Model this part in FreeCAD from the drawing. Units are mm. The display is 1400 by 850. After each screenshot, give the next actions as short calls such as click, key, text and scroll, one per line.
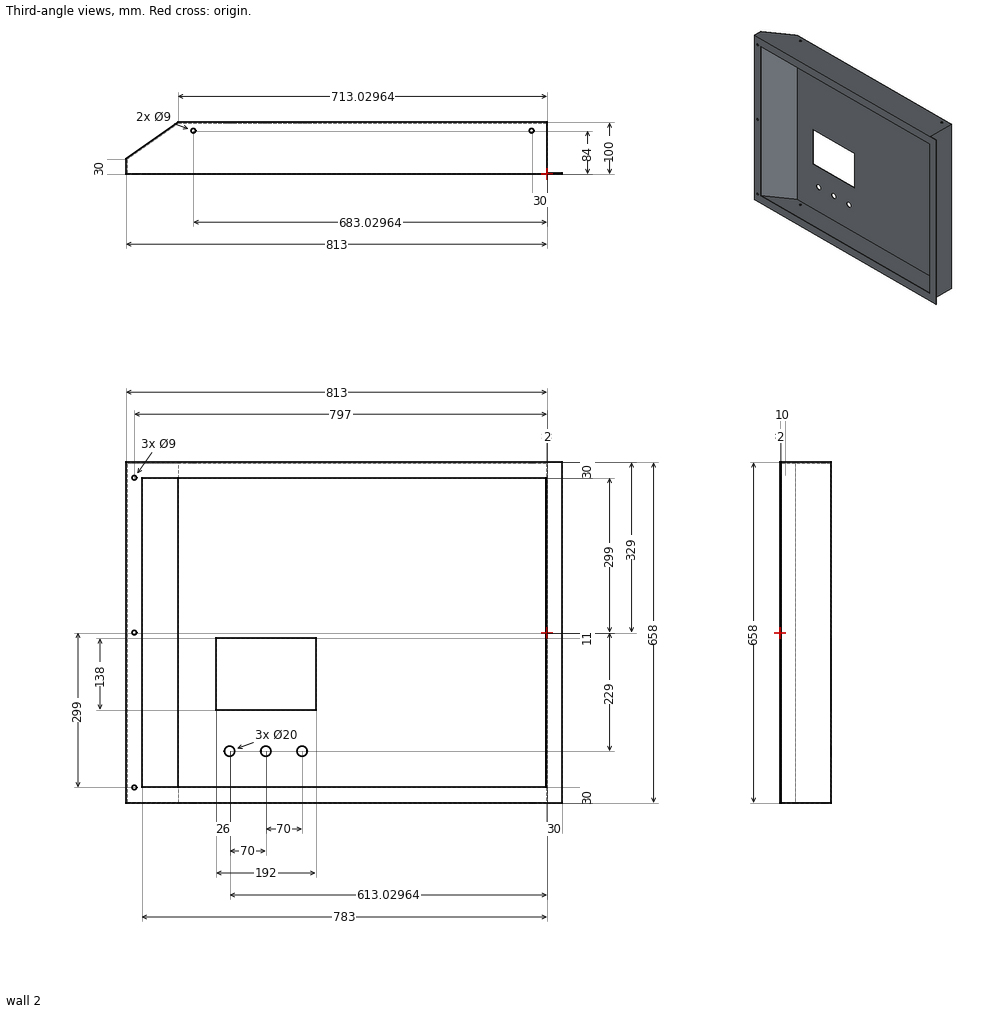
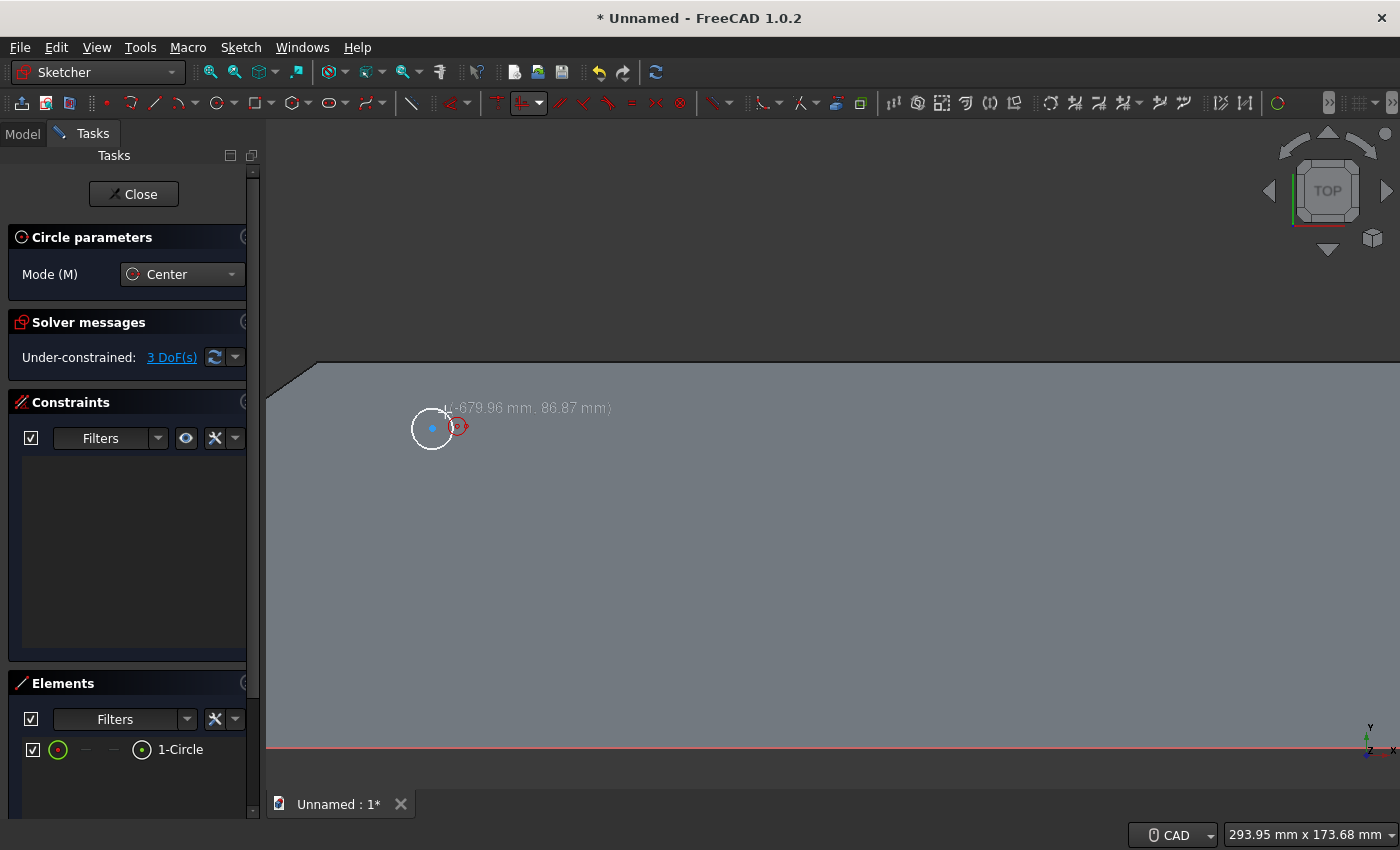
scroll(445, 414, down, 7)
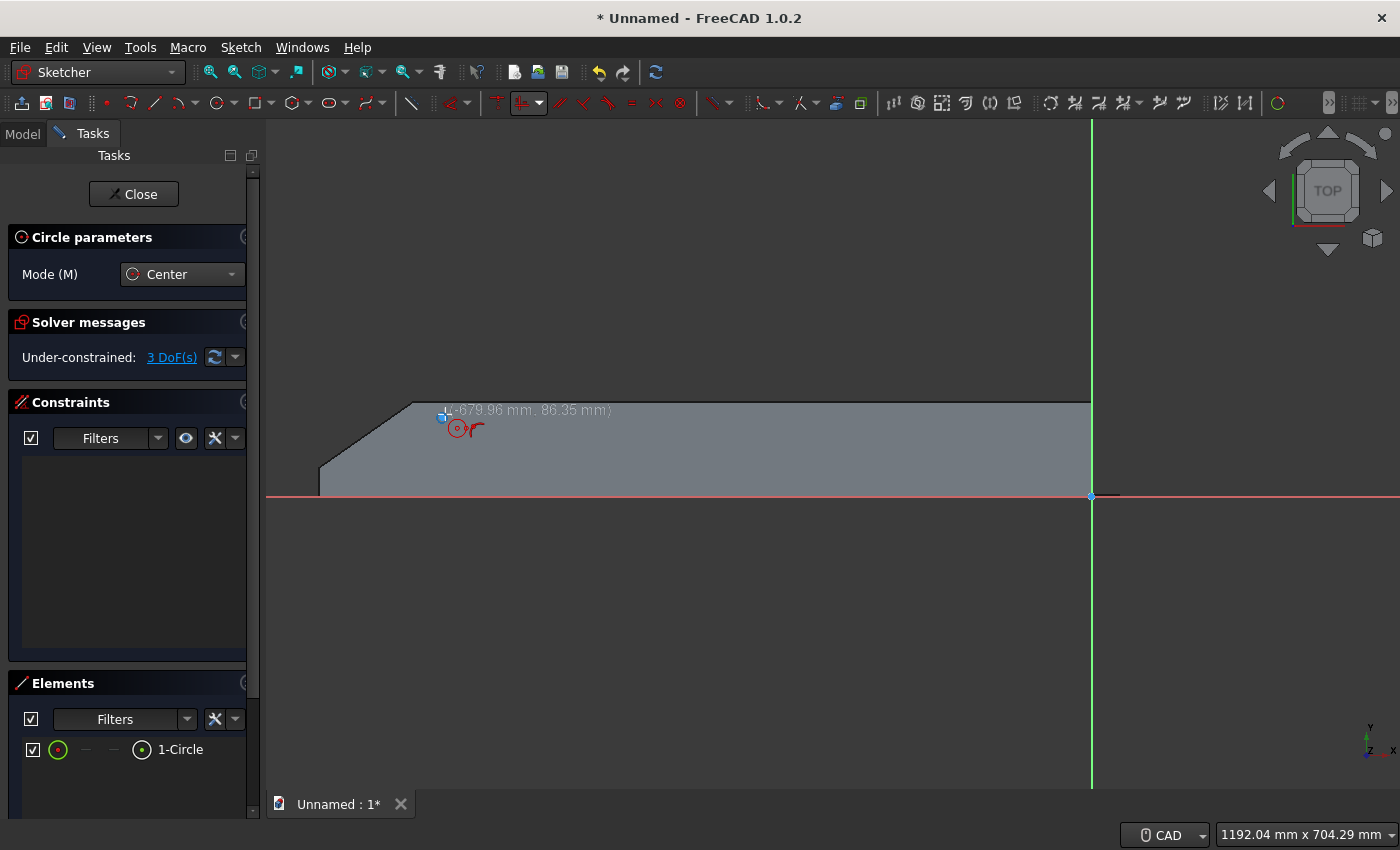
scroll(1063, 417, up, 9)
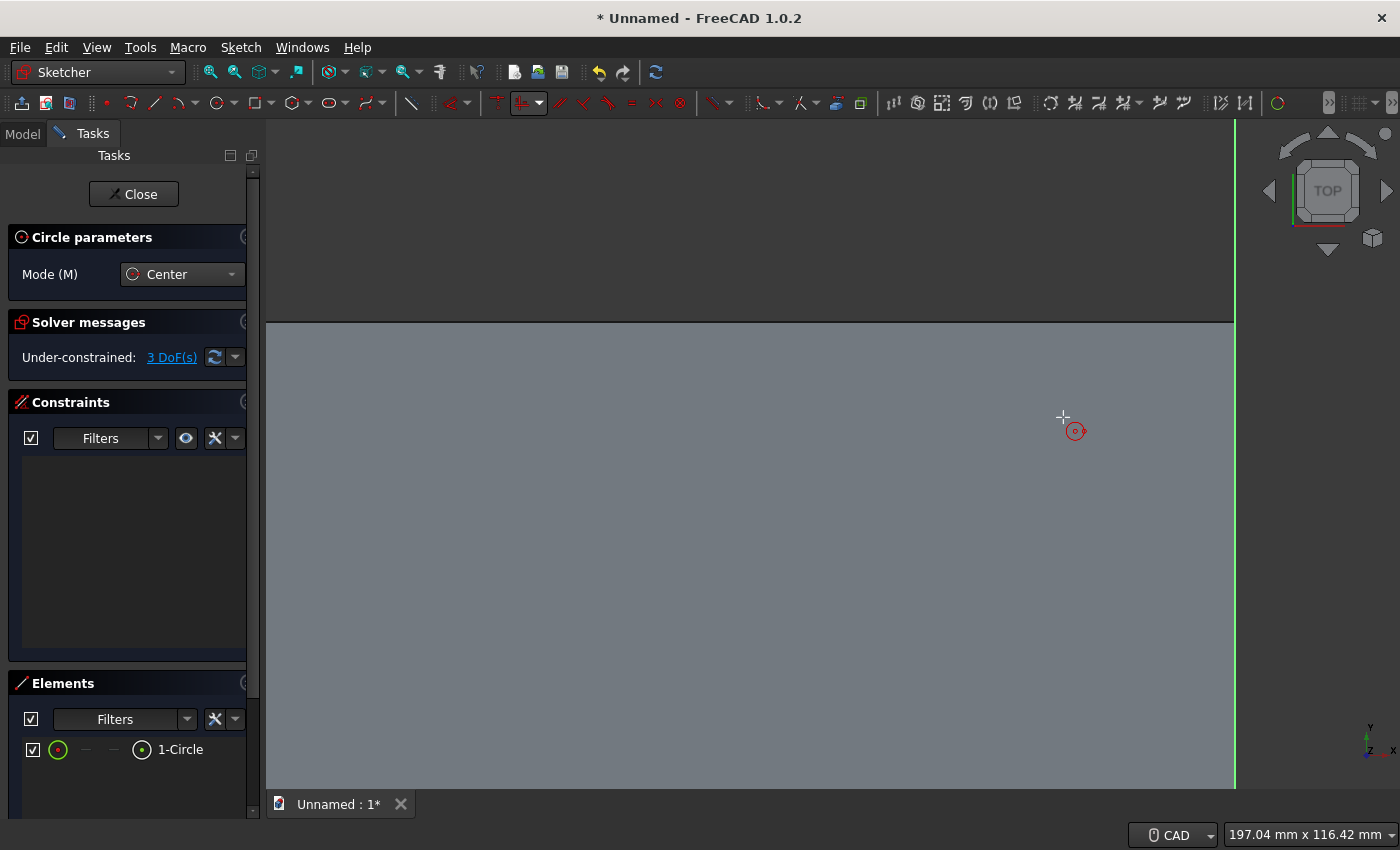
scroll(1063, 417, down, 9)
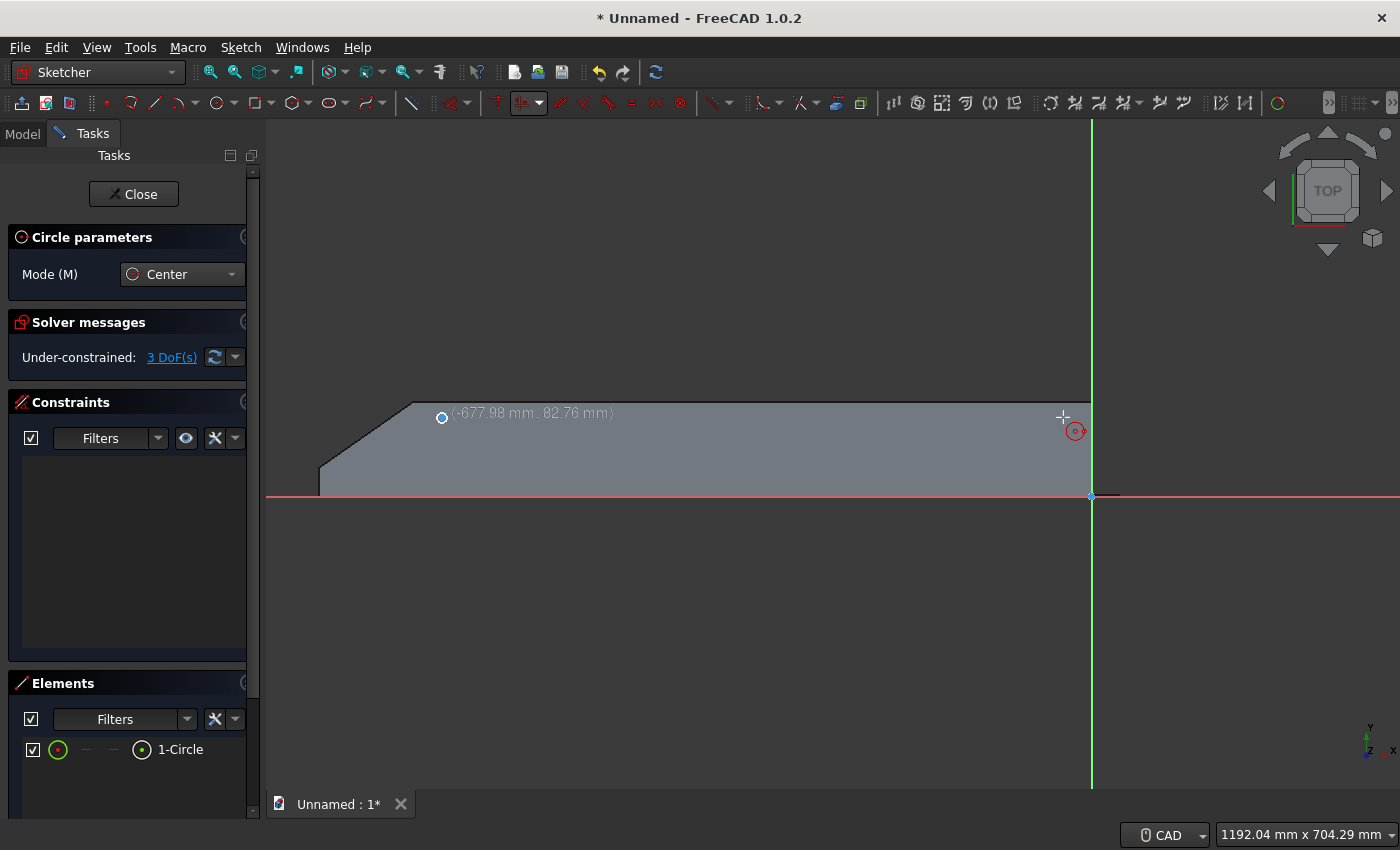
click(1063, 417)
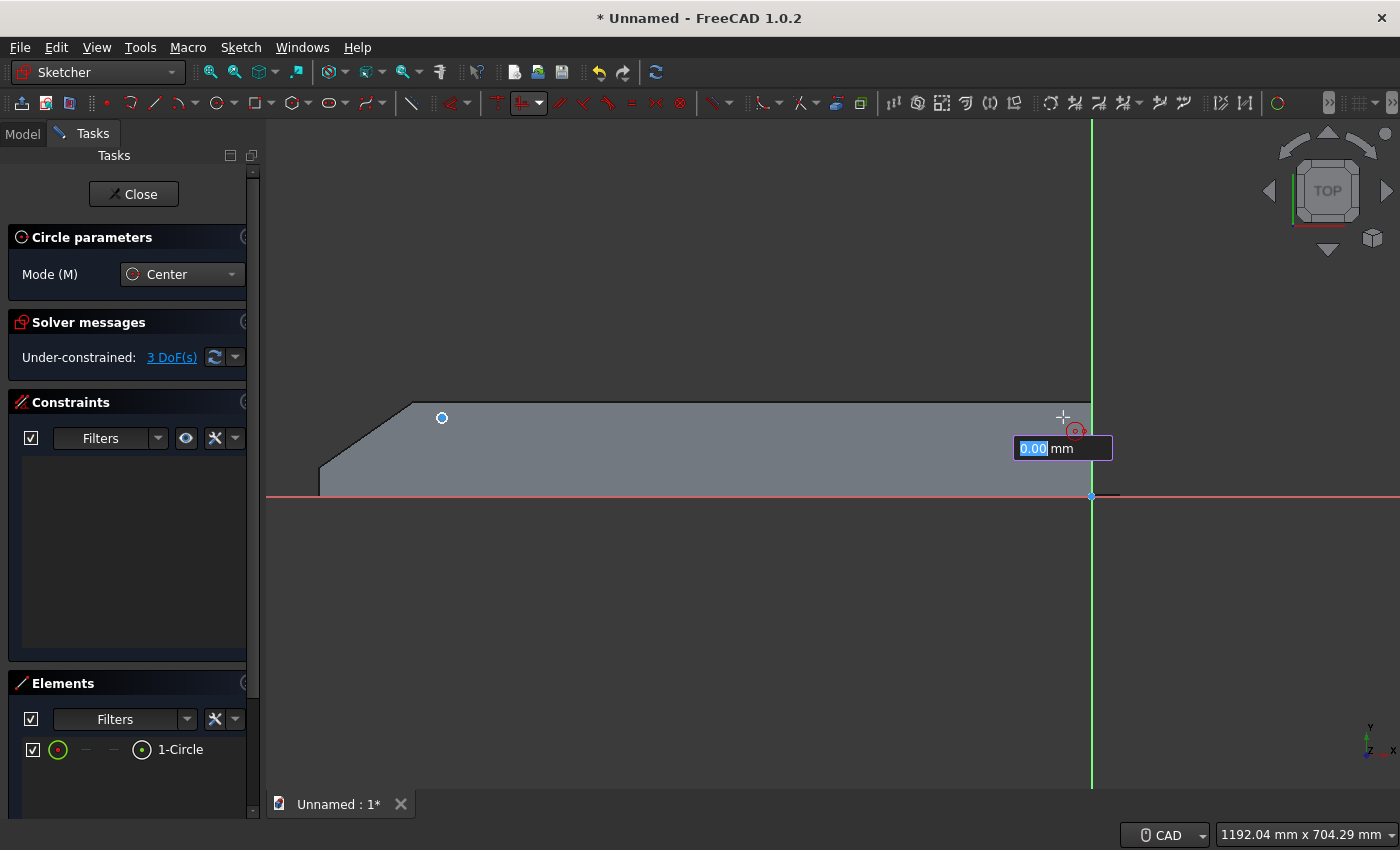
scroll(1066, 414, up, 7)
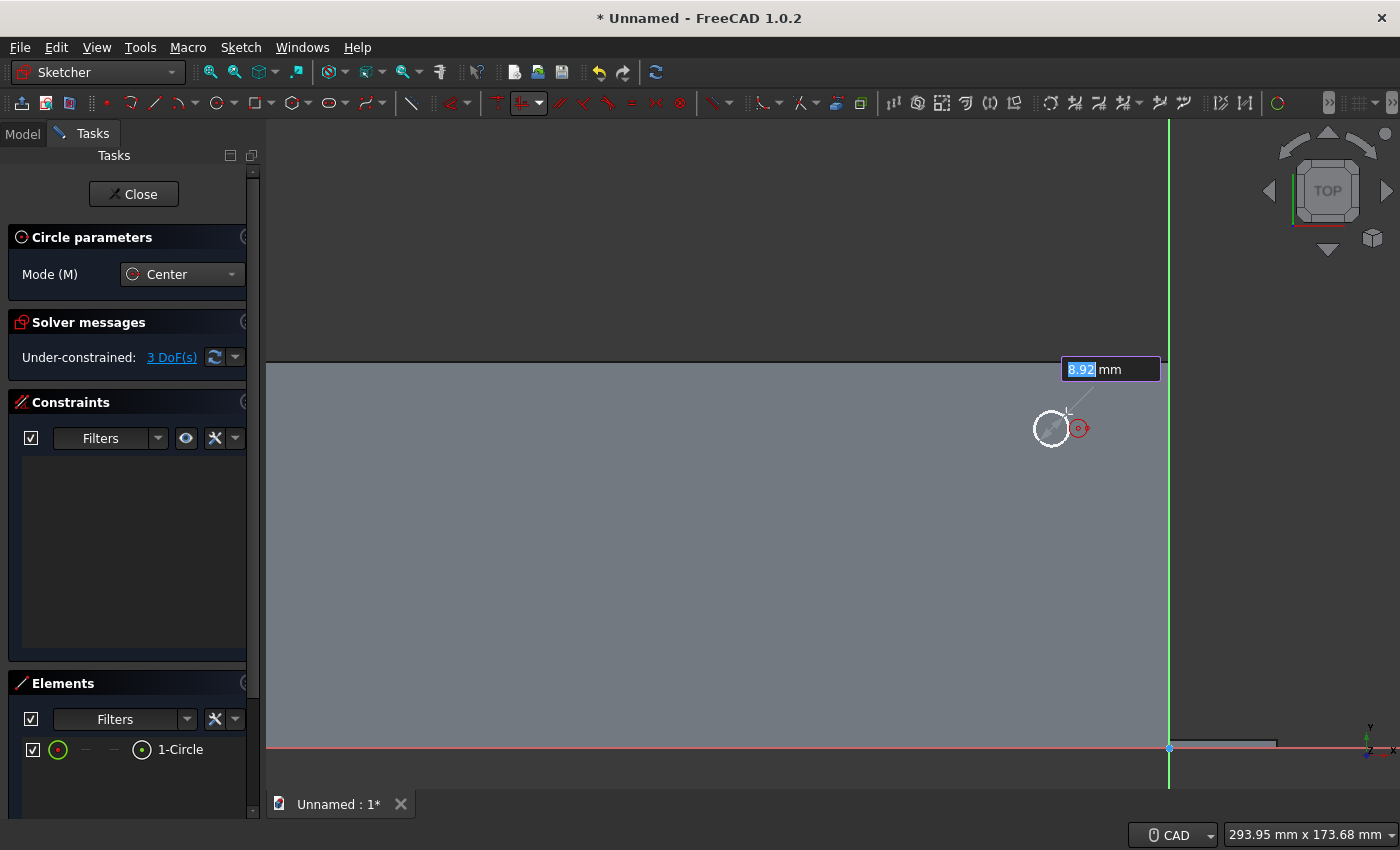
click(1066, 412)
key(Escape)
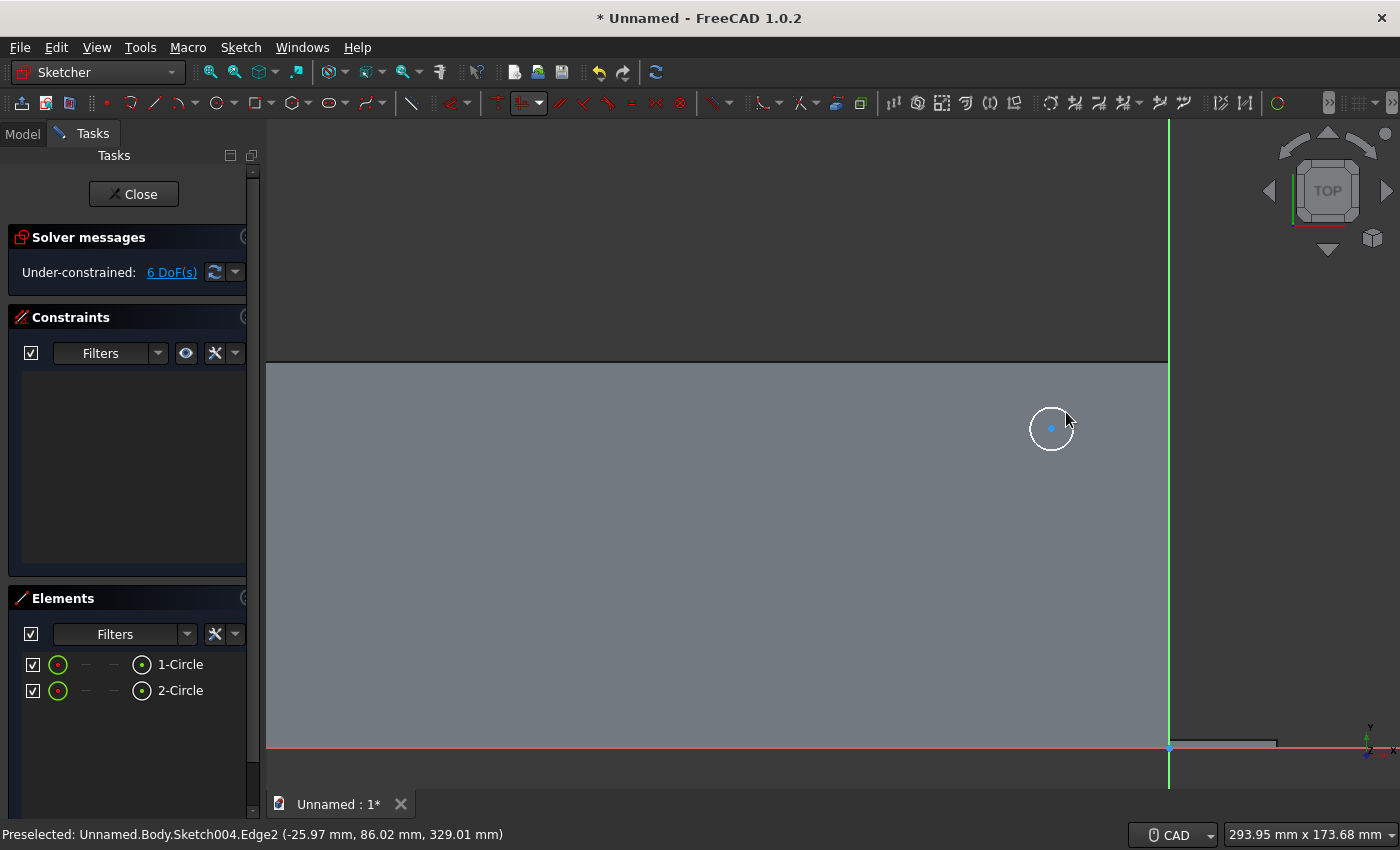
scroll(1066, 414, down, 7)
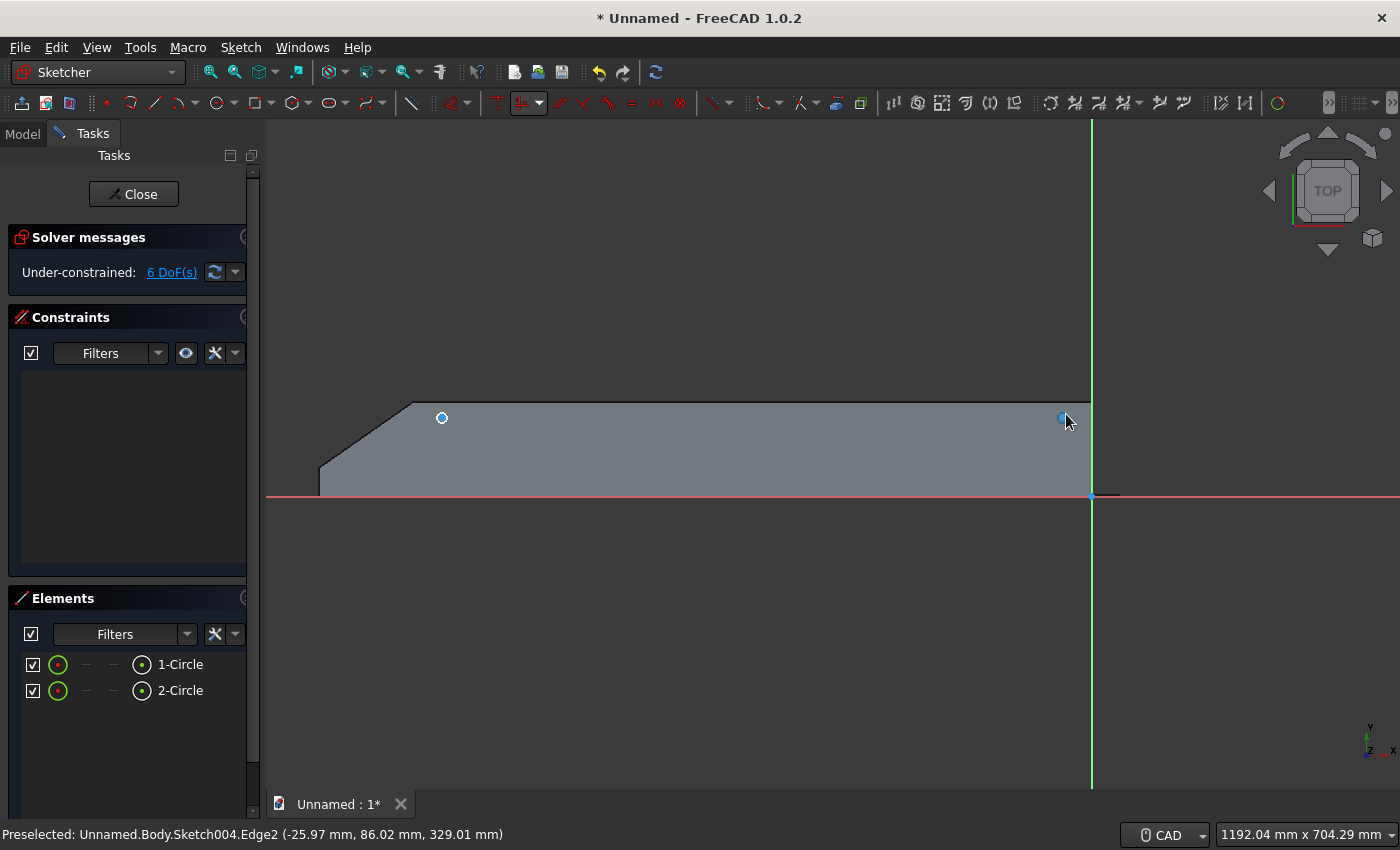
scroll(446, 414, up, 6)